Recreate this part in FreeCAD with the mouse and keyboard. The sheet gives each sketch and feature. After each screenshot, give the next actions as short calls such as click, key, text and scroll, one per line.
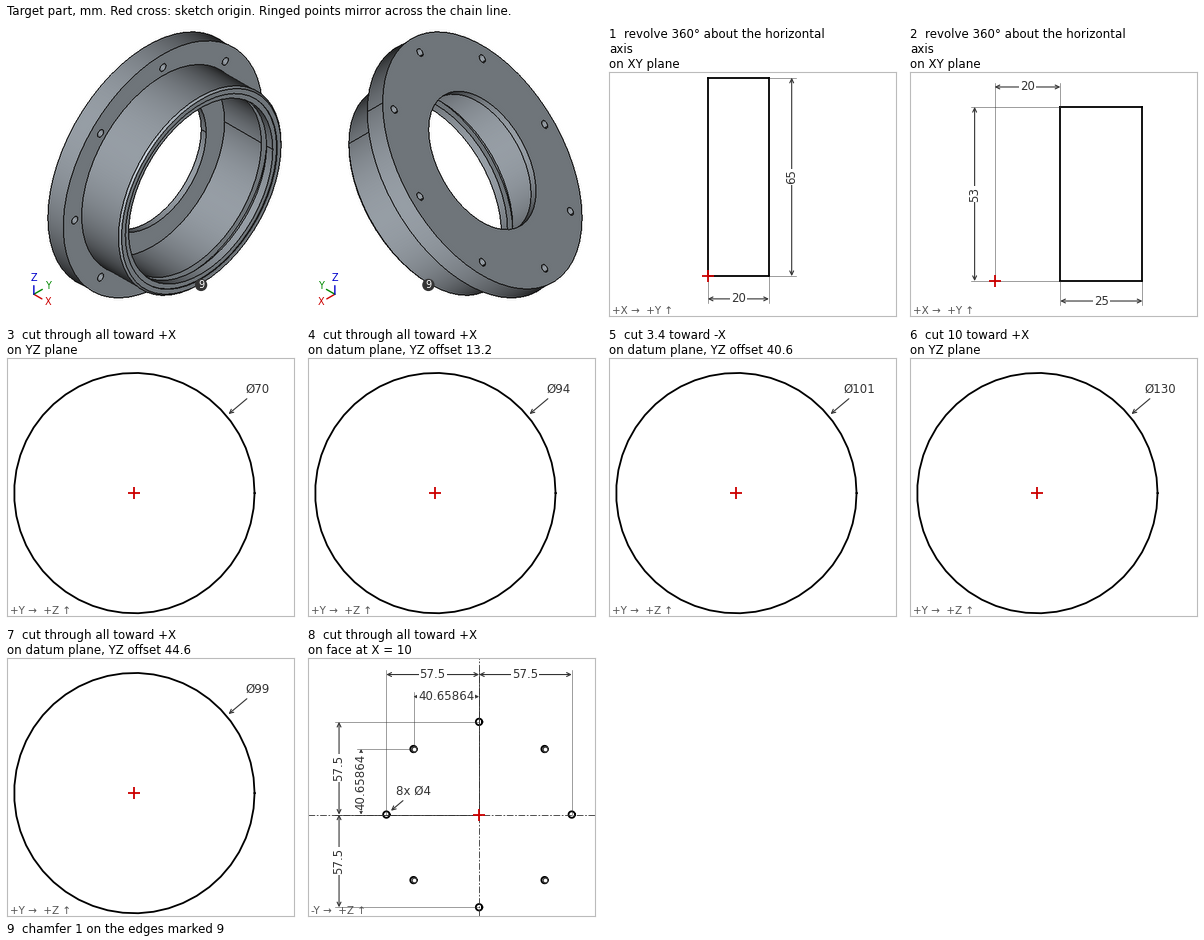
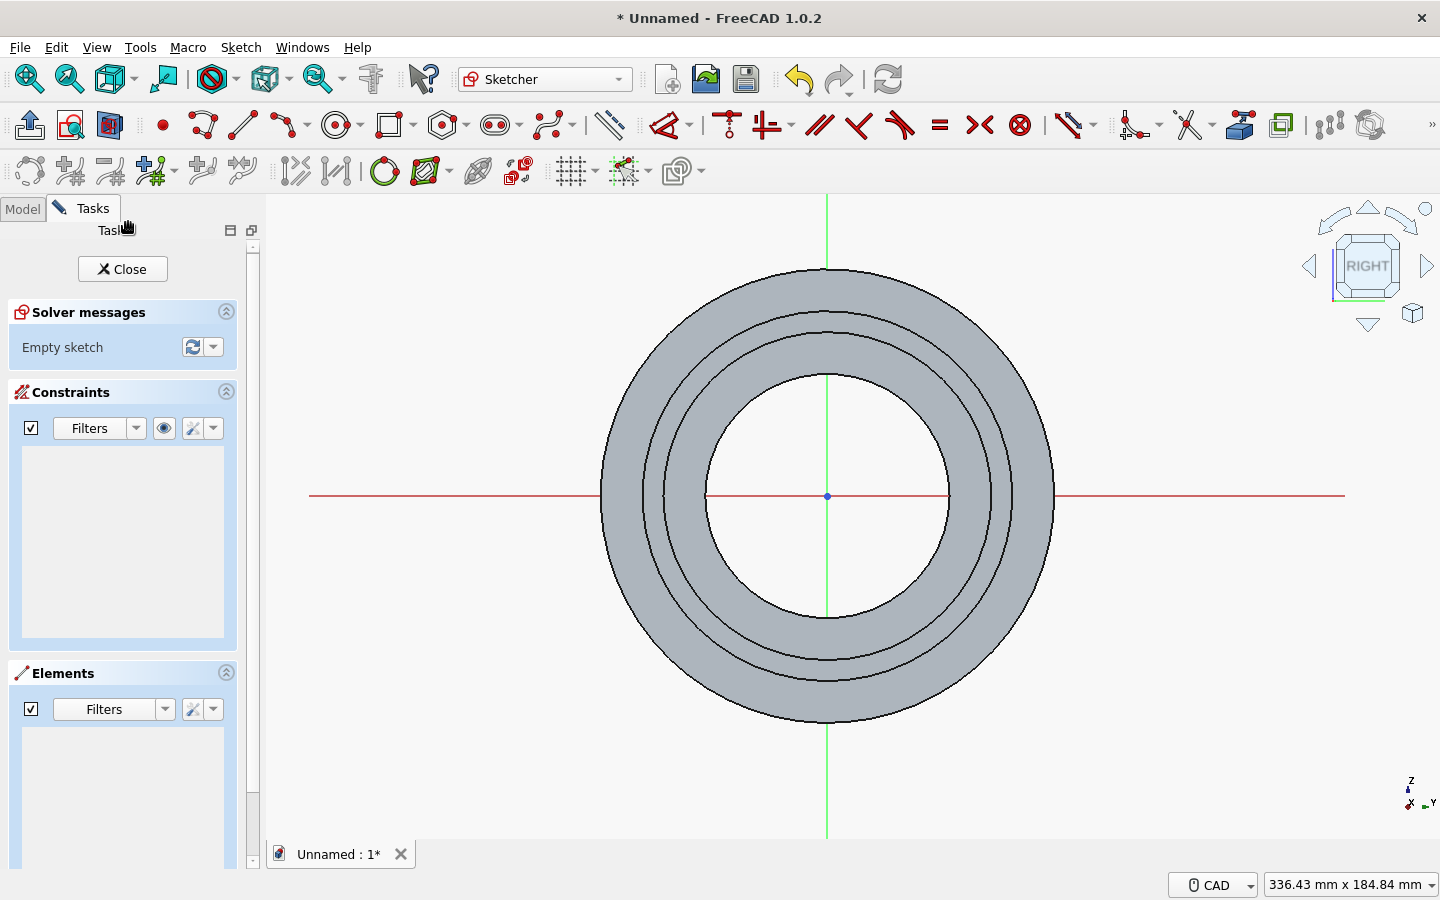
click(110, 126)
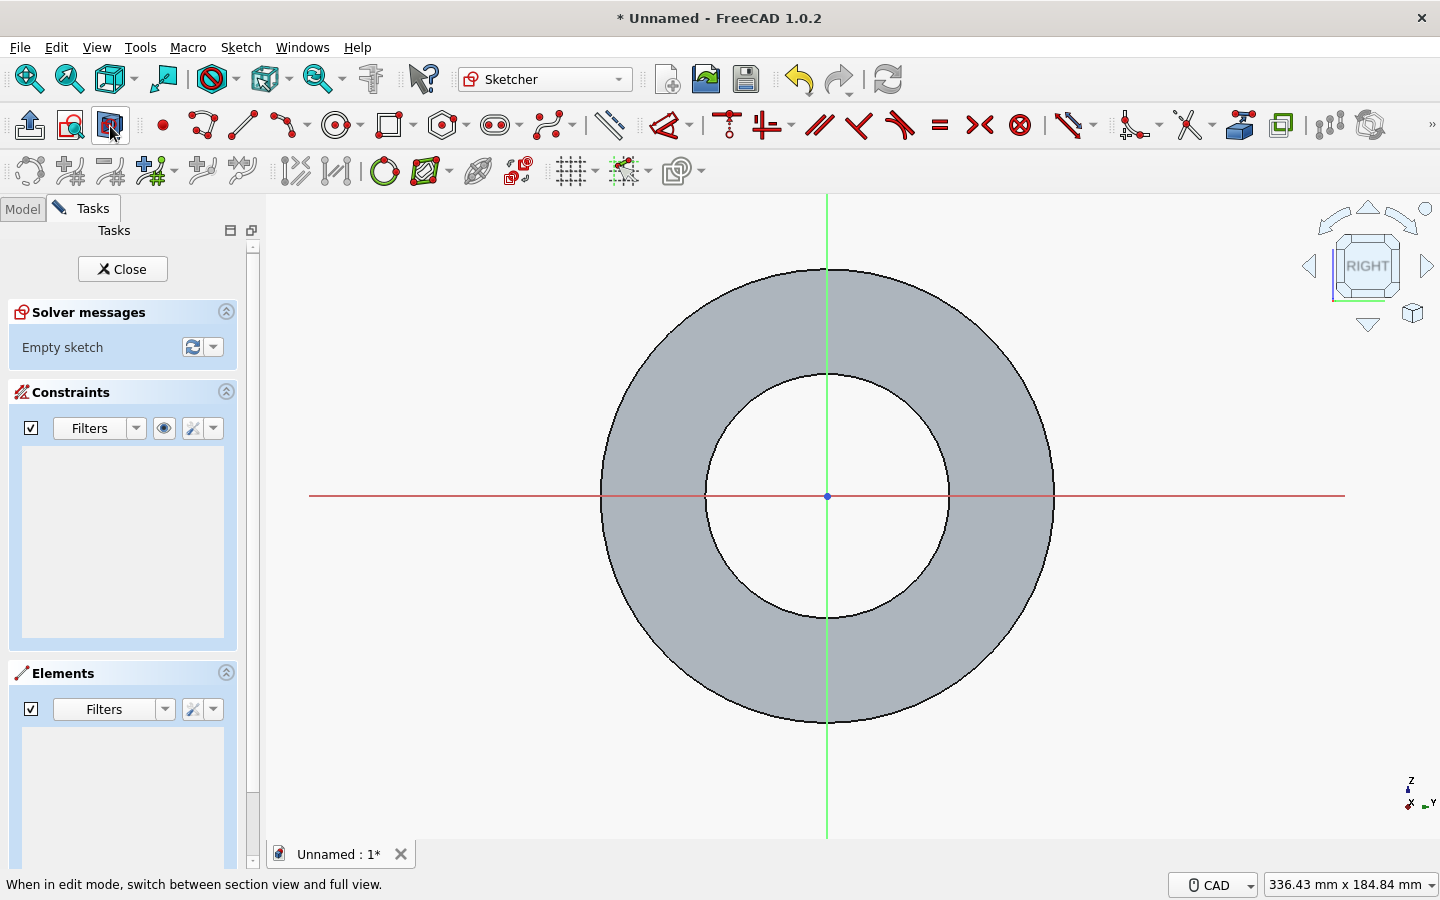
click(336, 126)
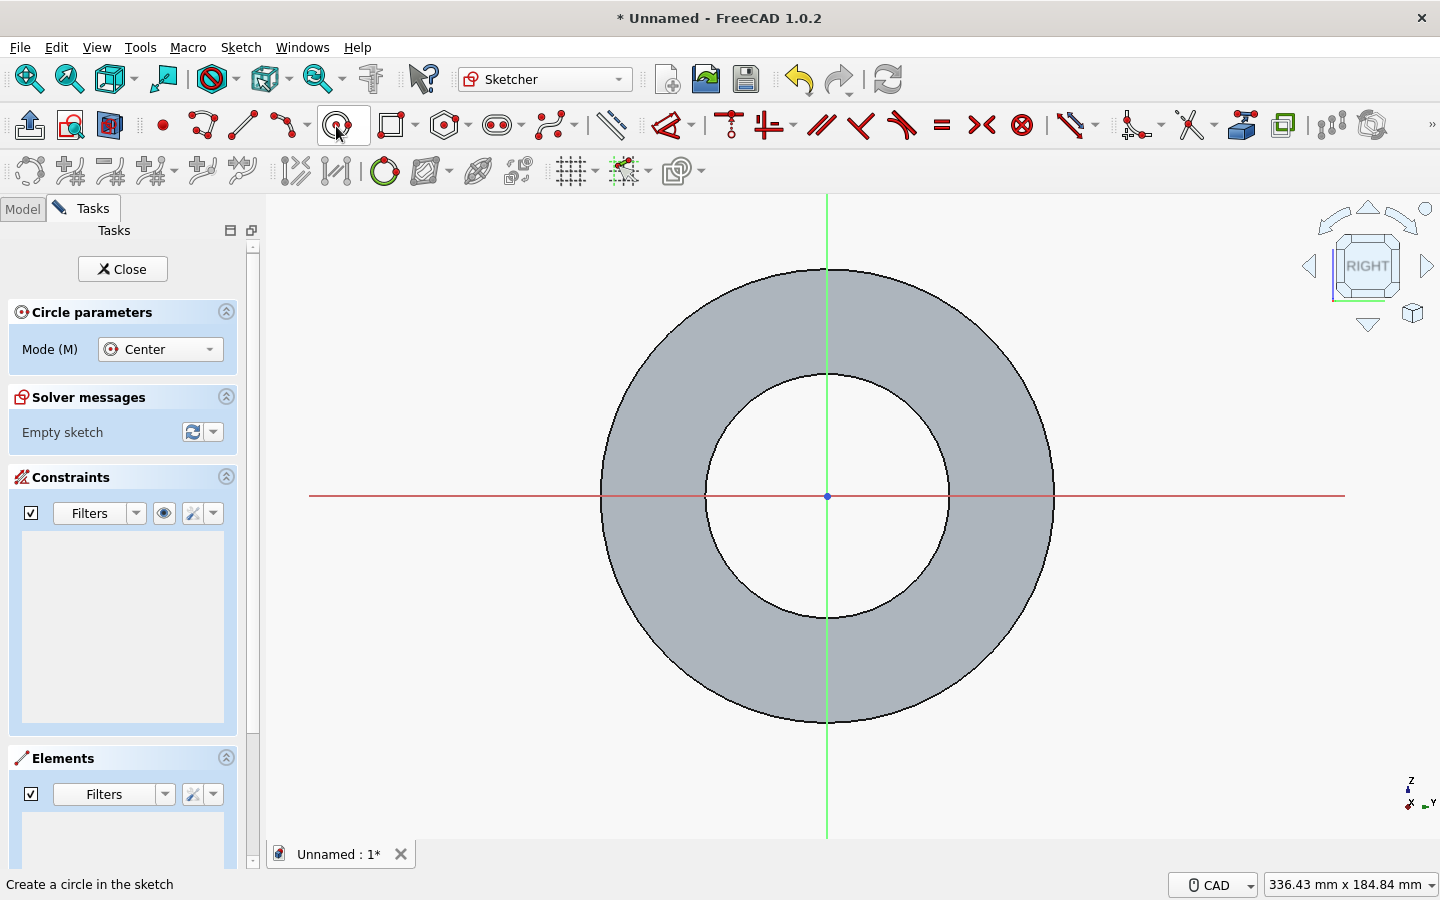
click(827, 496)
click(988, 336)
key(Escape)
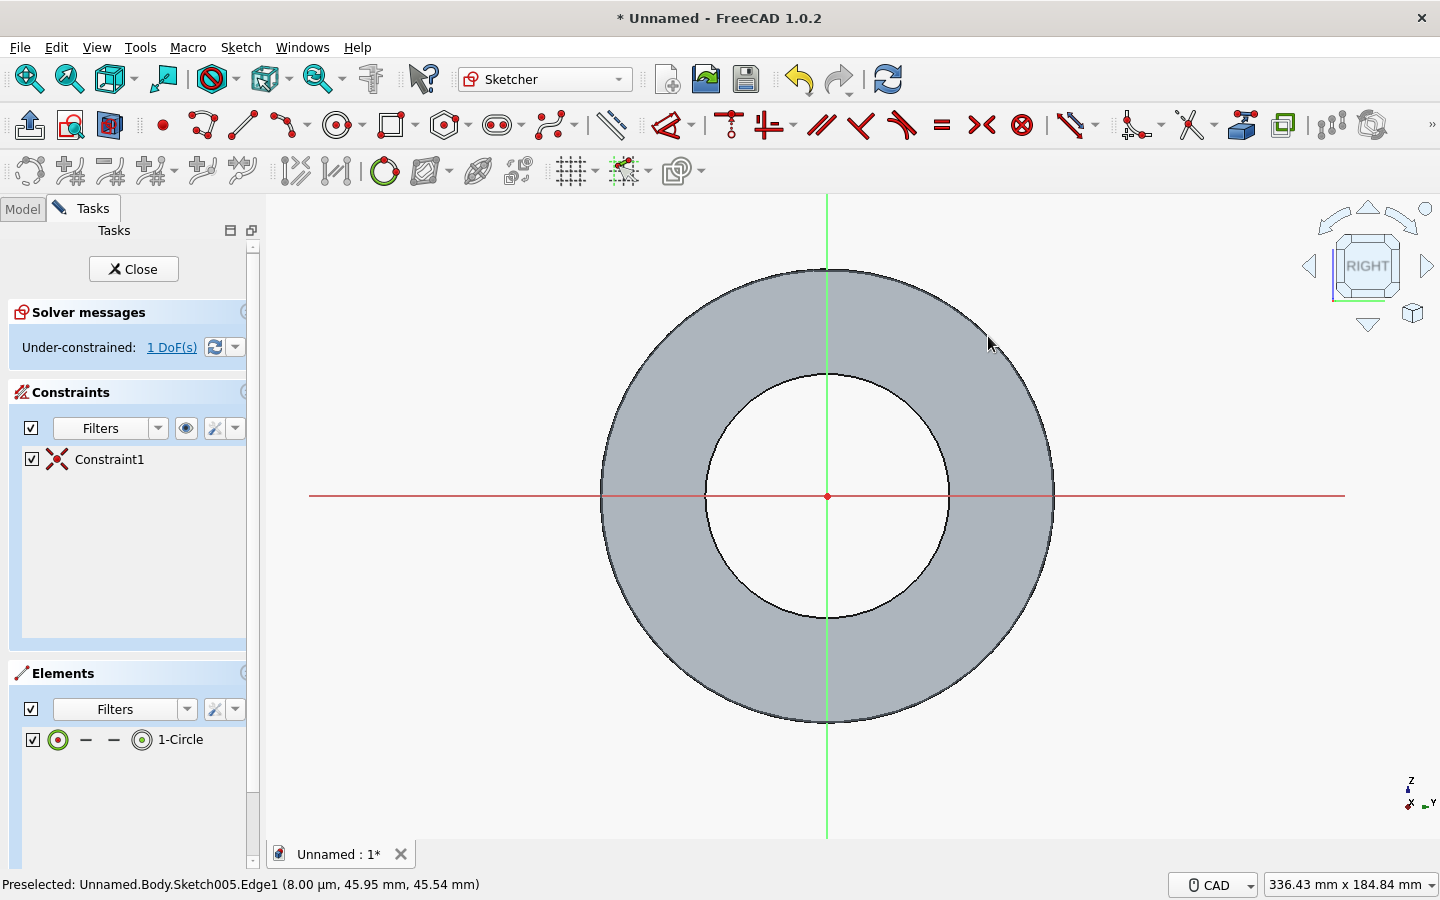
click(666, 126)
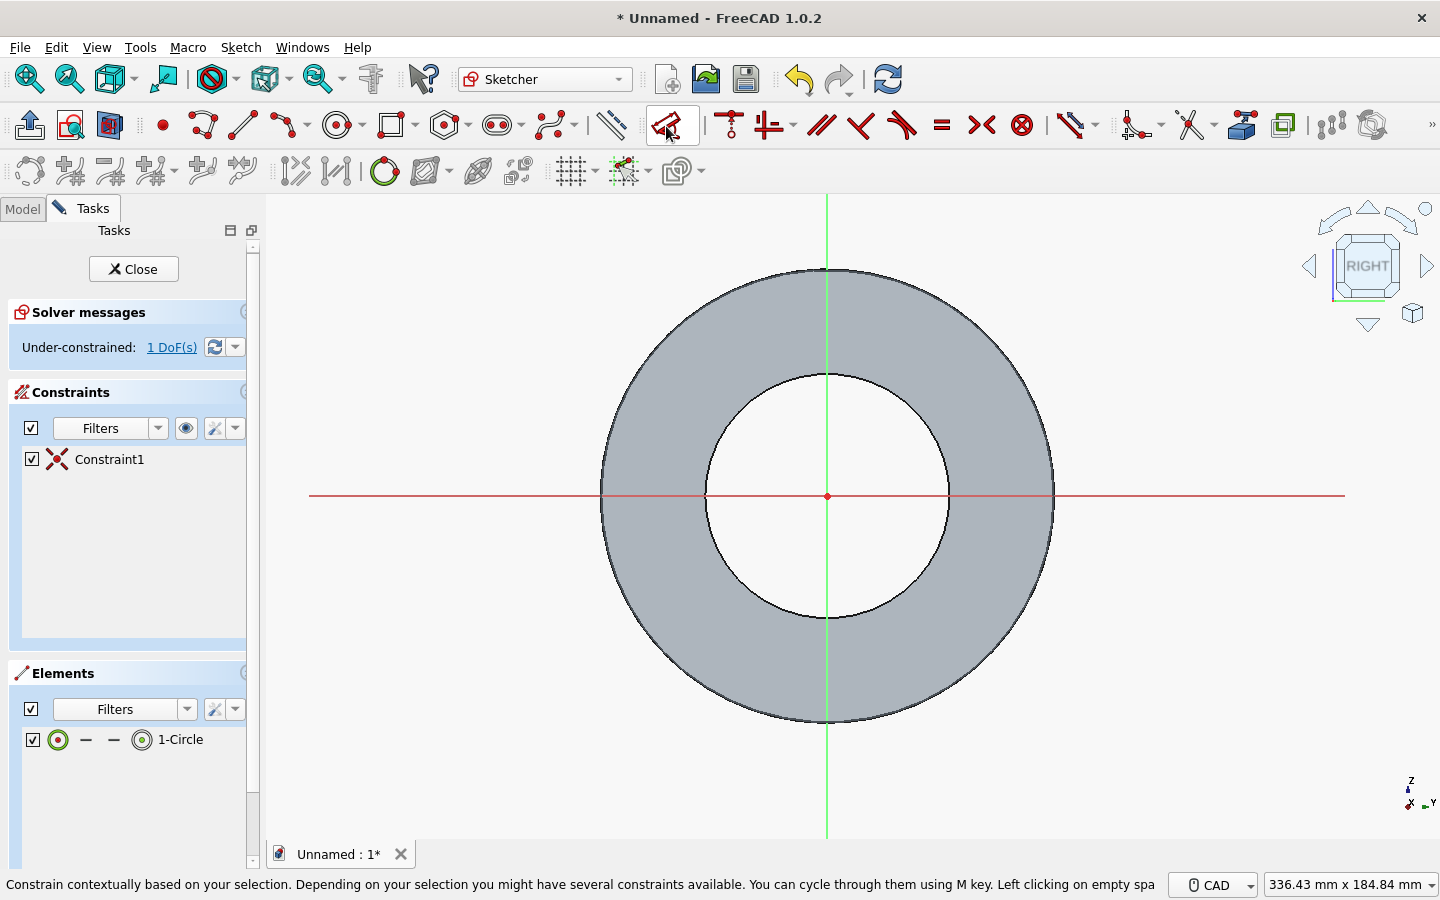
click(987, 336)
click(1010, 313)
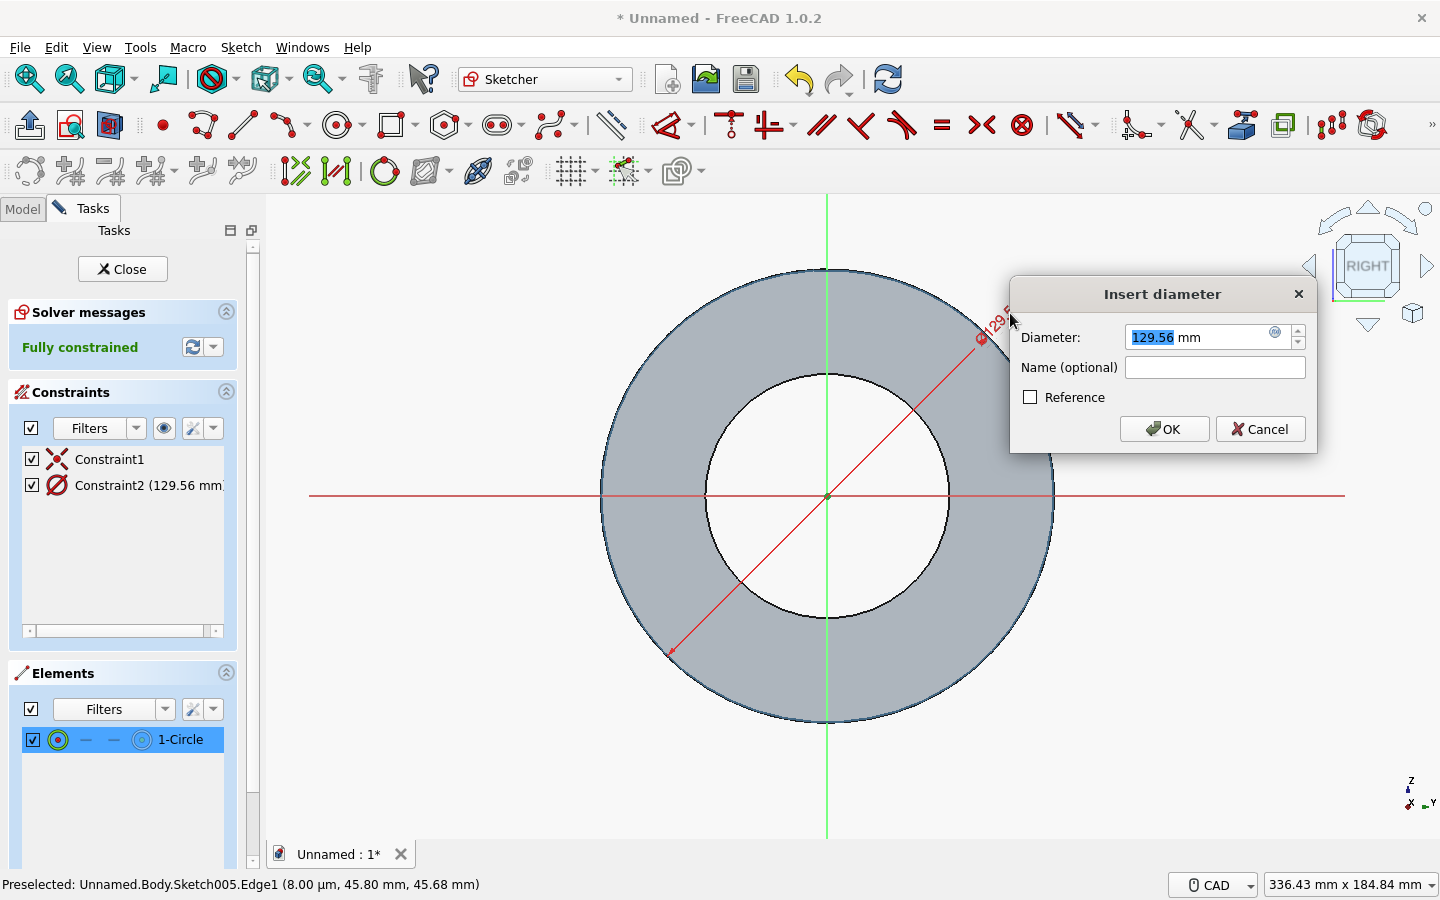
text(130)
key(Return)
key(Escape)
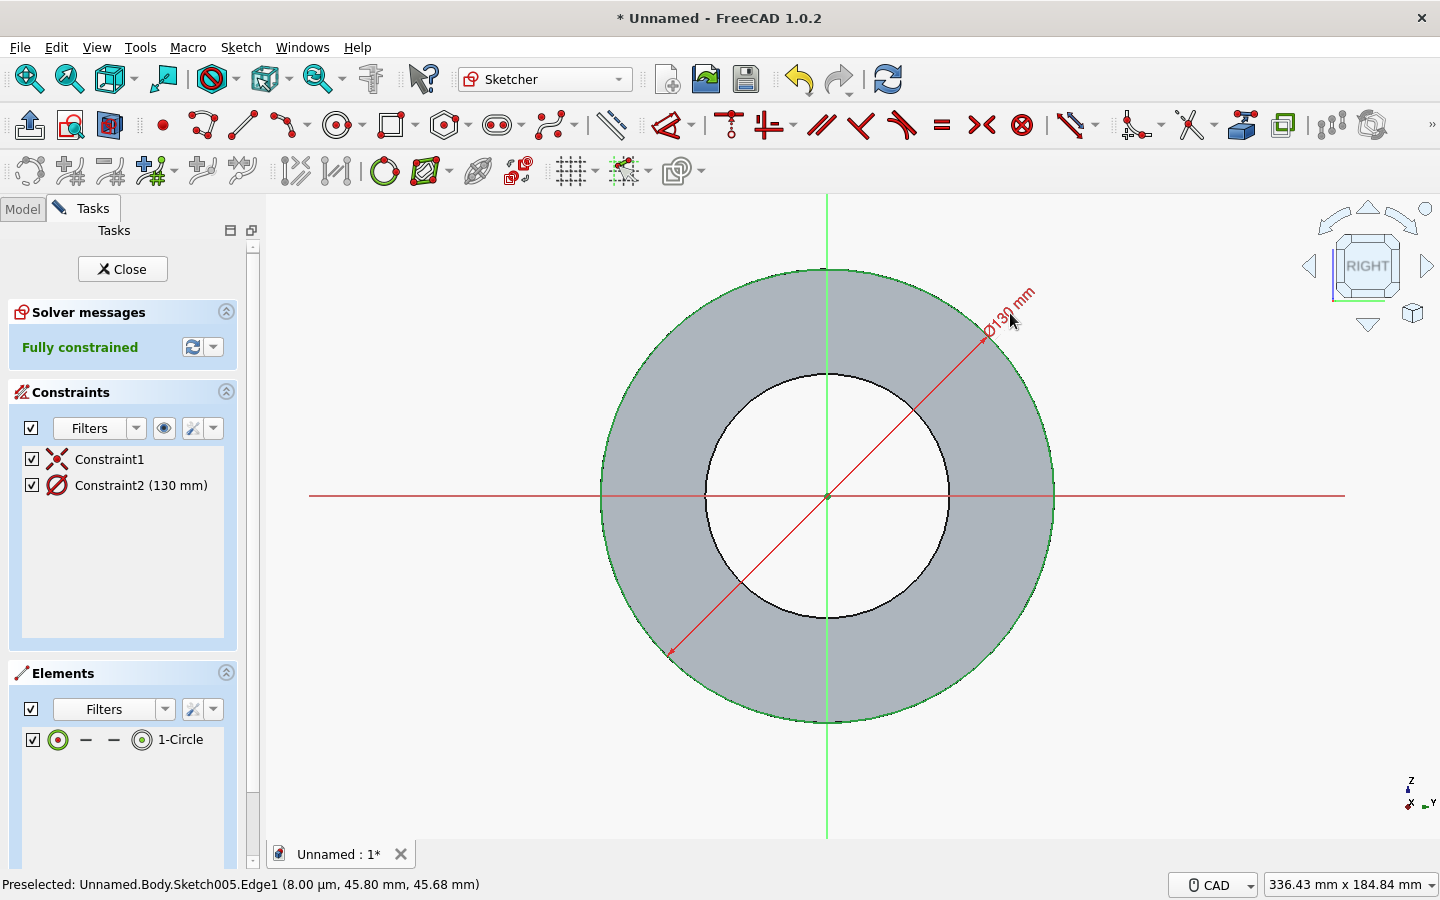
click(123, 269)